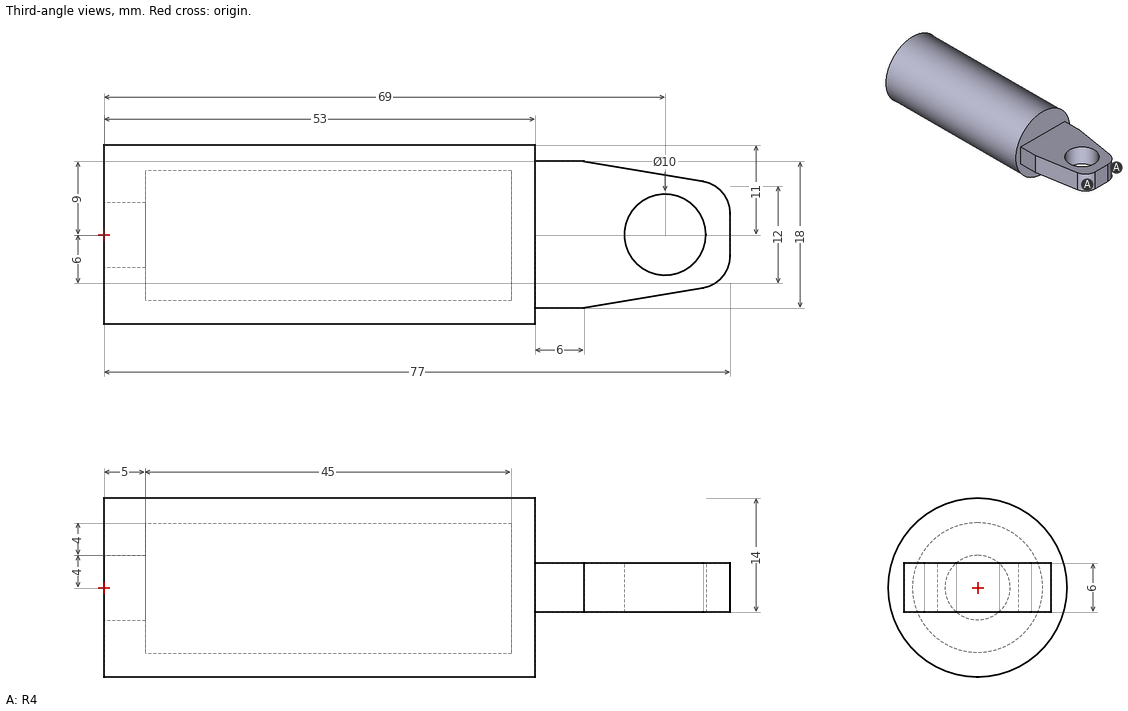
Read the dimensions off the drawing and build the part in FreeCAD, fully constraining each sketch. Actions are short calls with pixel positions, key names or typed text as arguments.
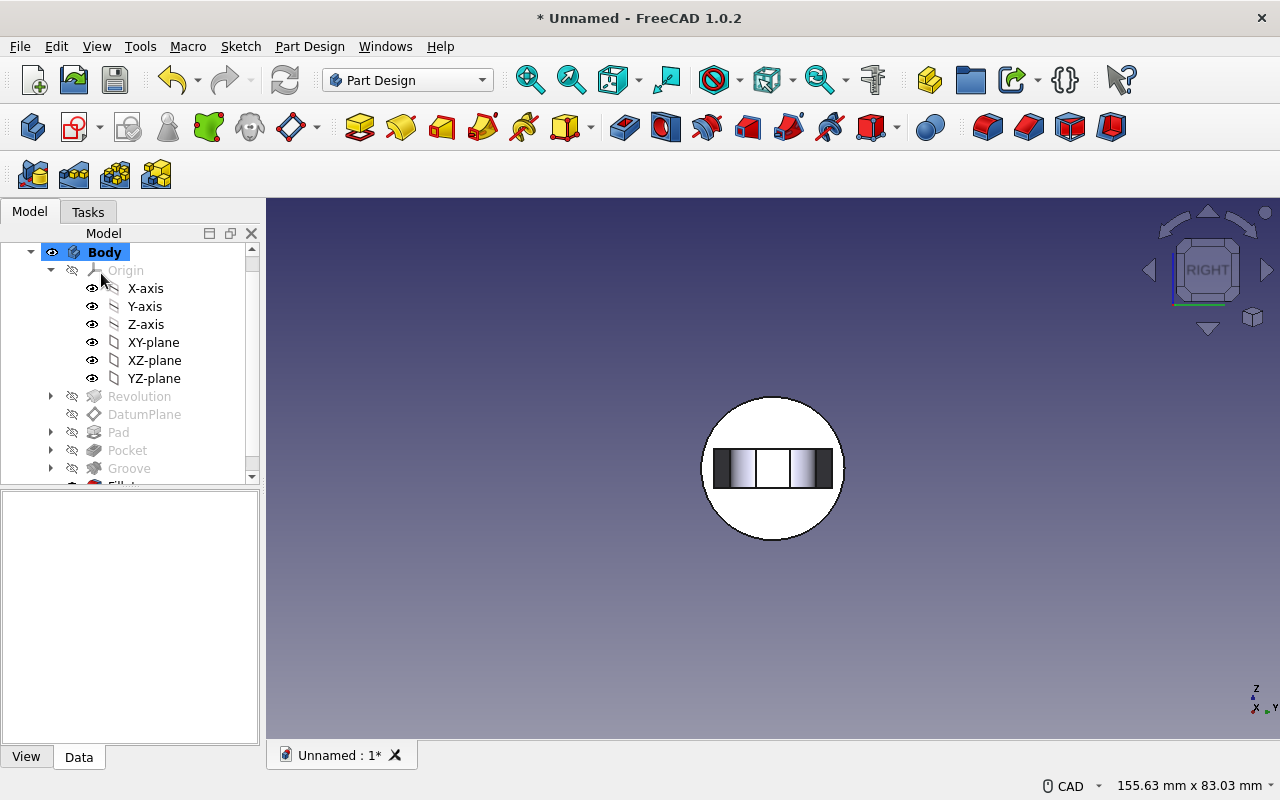
key(0)